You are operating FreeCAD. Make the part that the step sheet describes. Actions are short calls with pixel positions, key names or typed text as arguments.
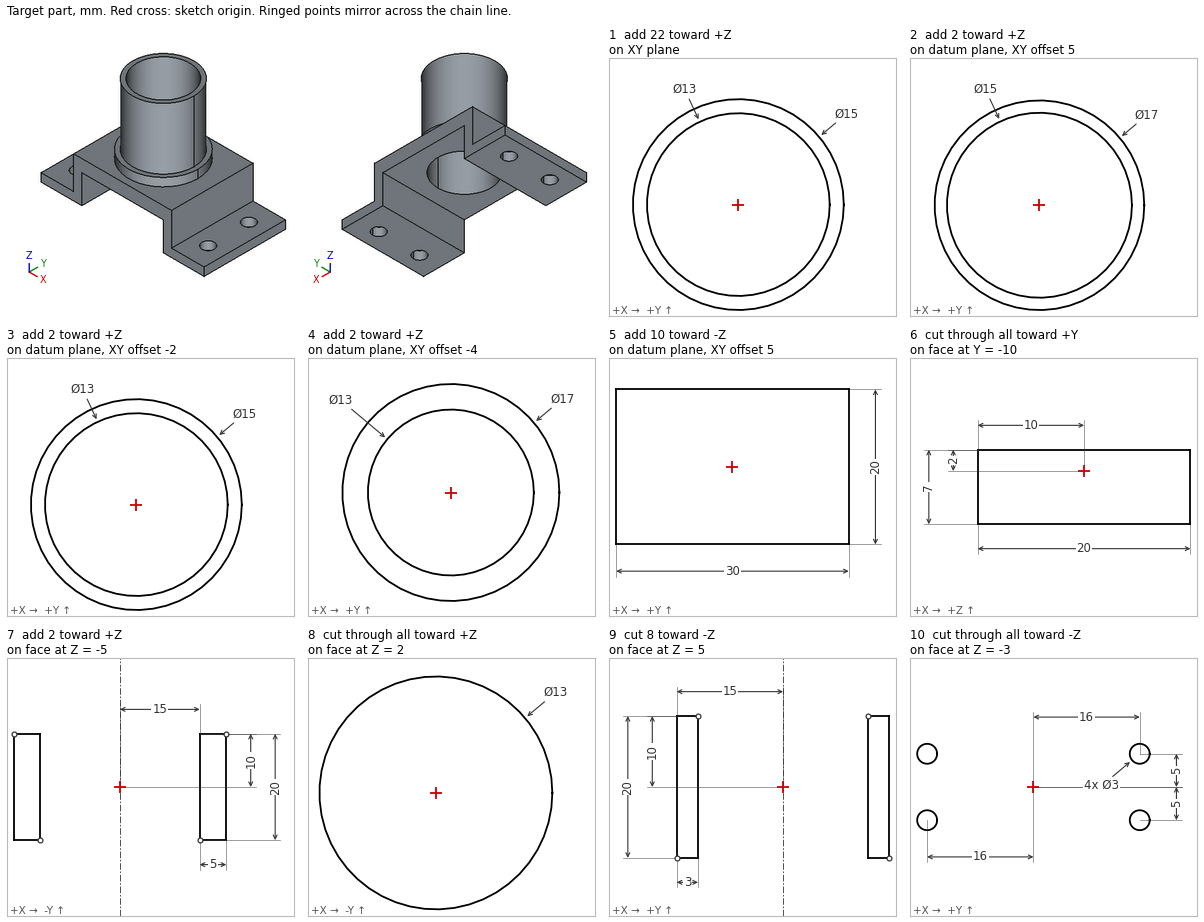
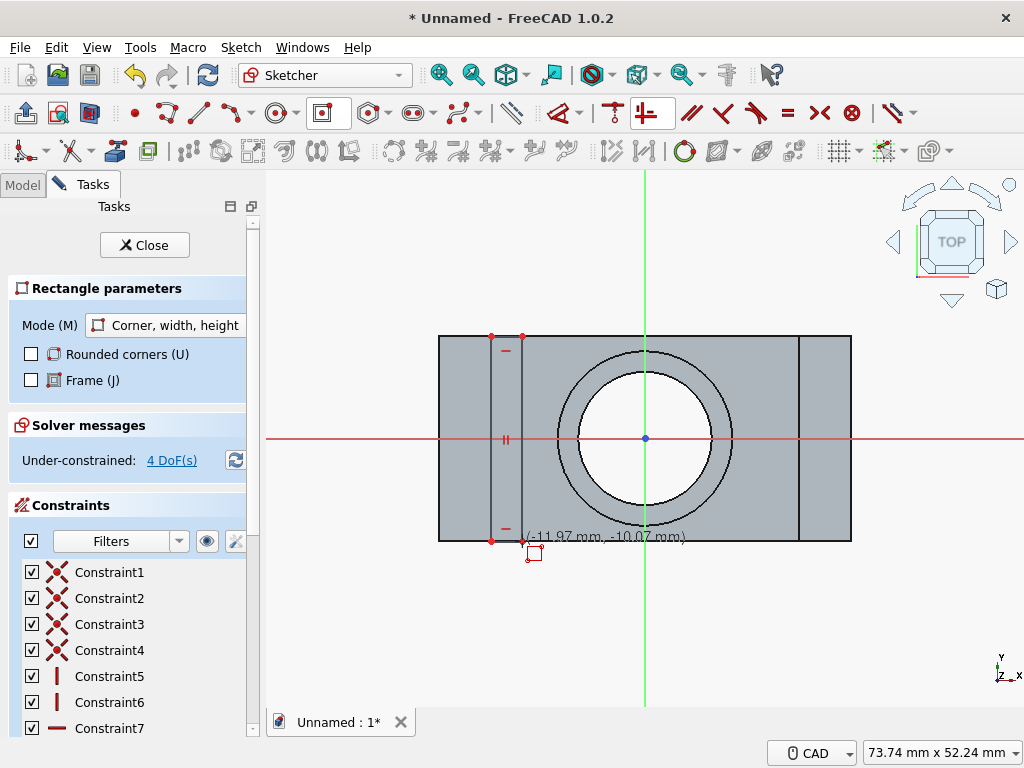
click(768, 336)
click(799, 541)
key(Escape)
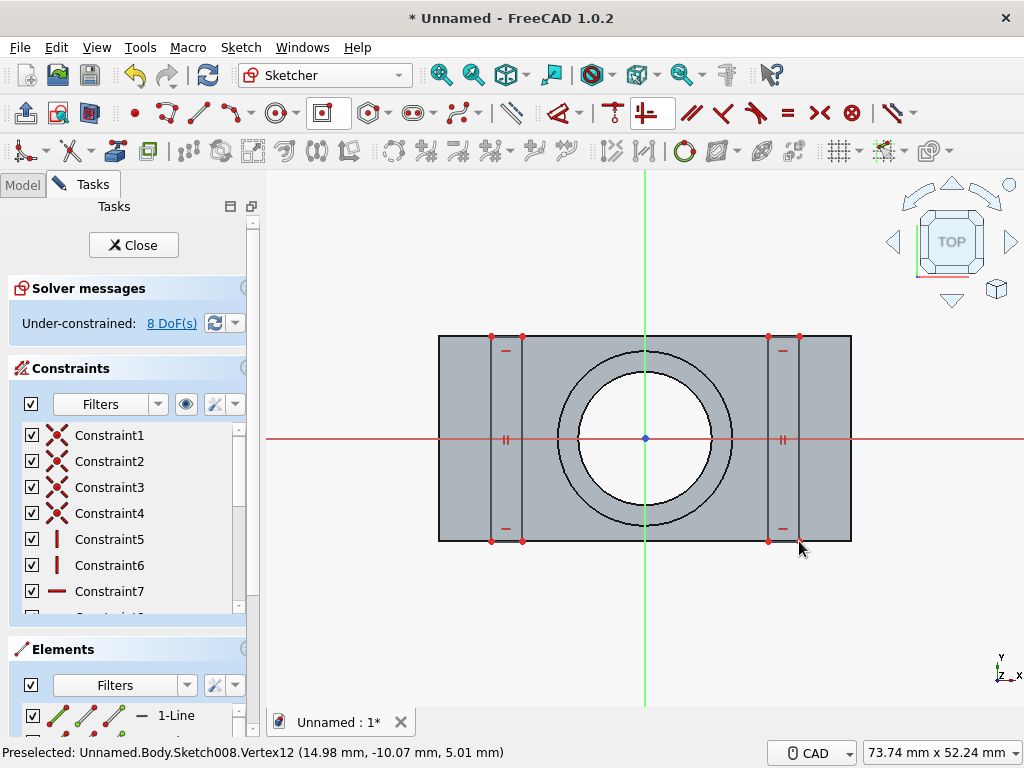
click(522, 337)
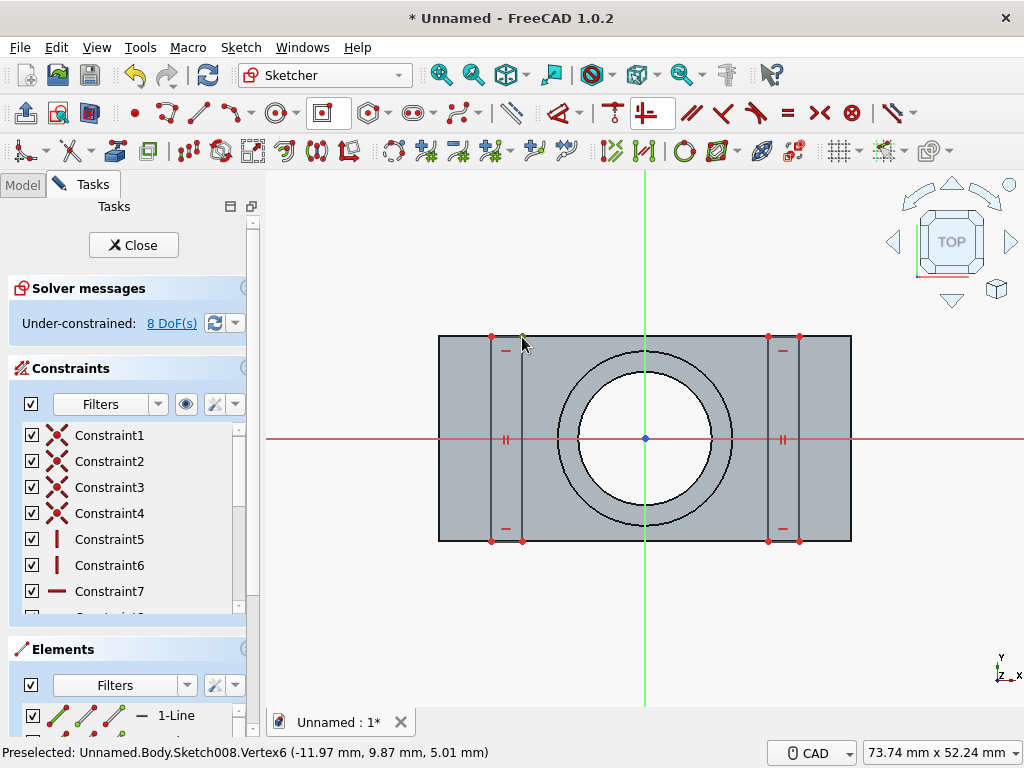
click(768, 337)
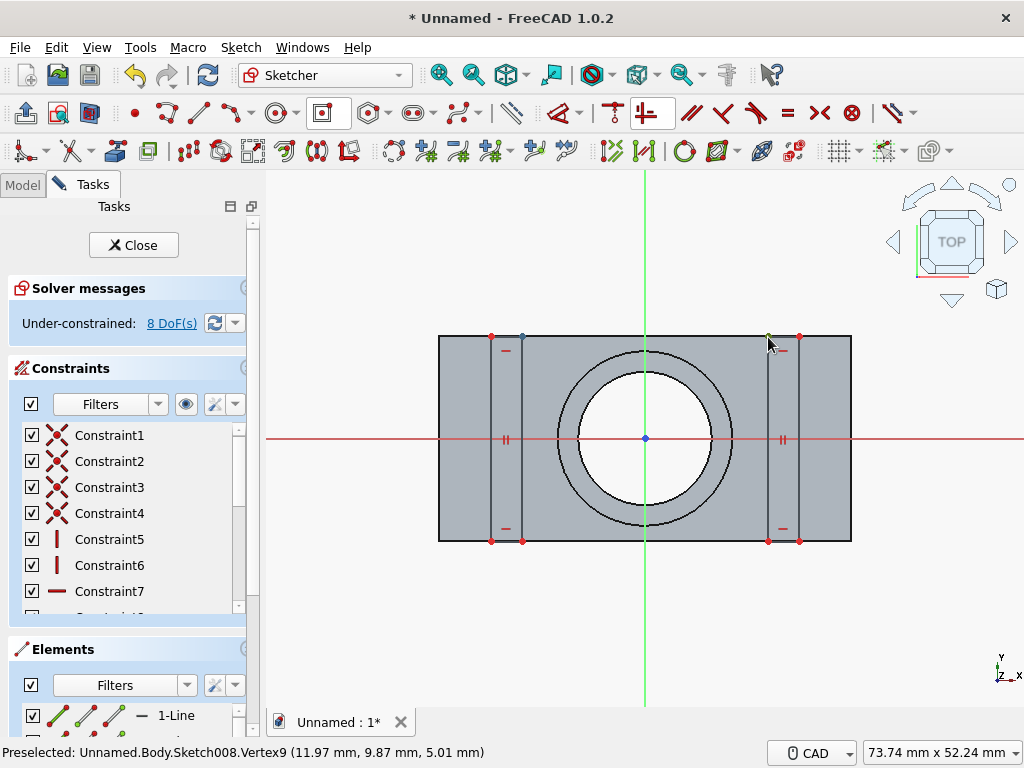
click(645, 645)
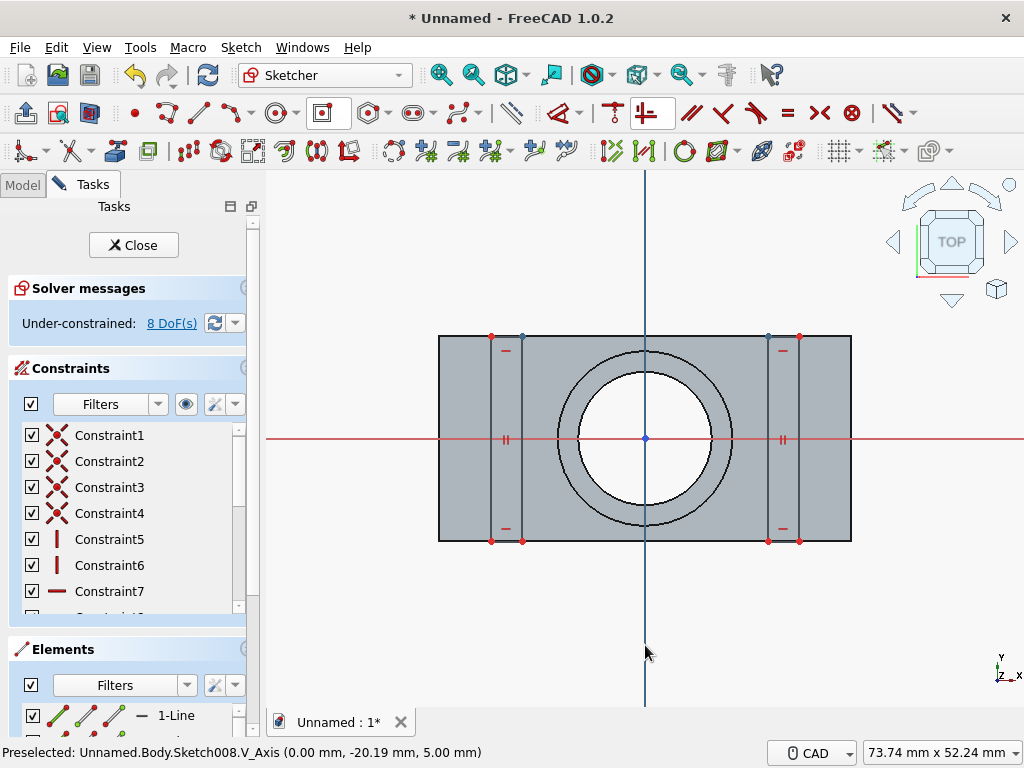
click(820, 114)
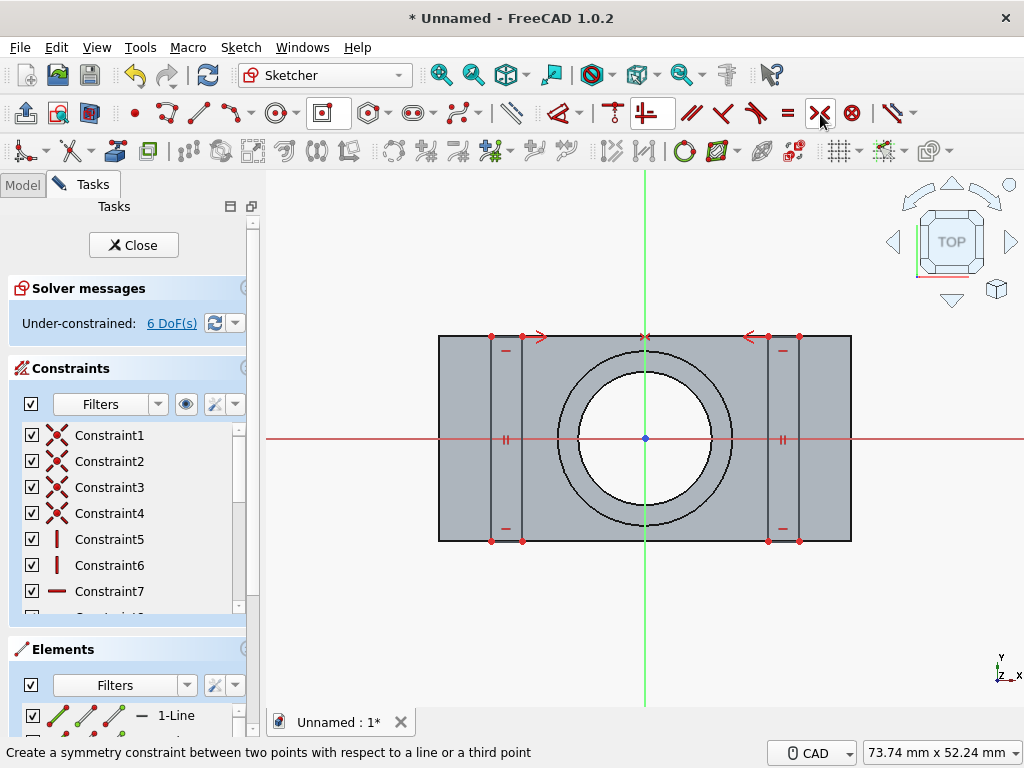
click(491, 542)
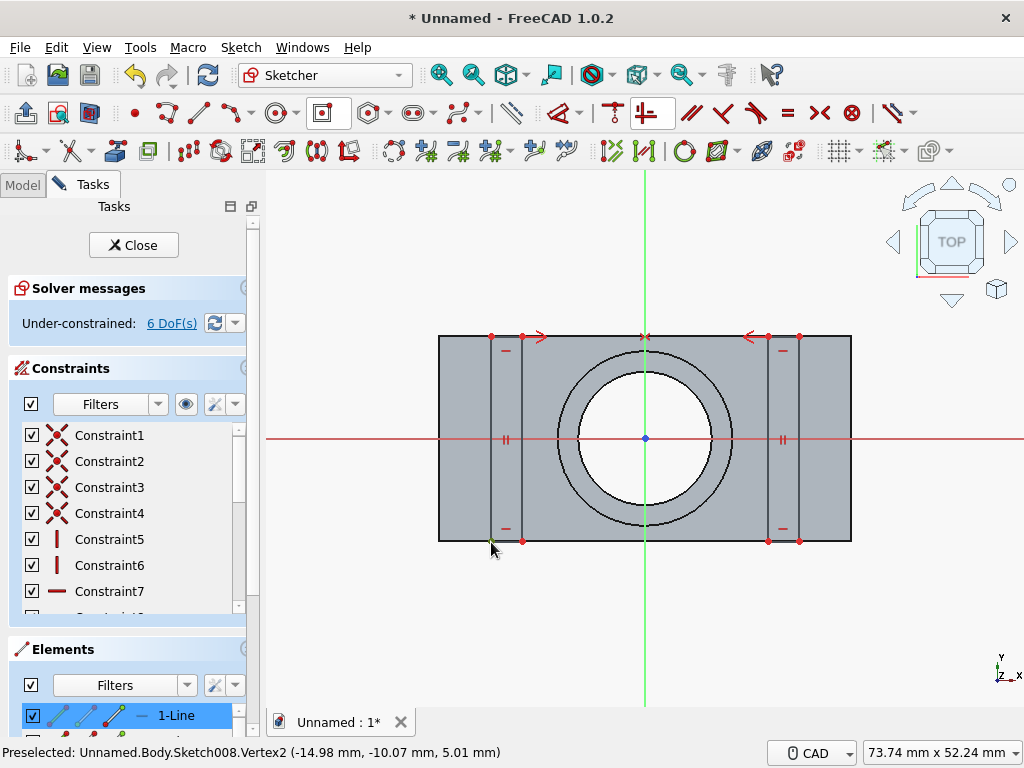
click(799, 542)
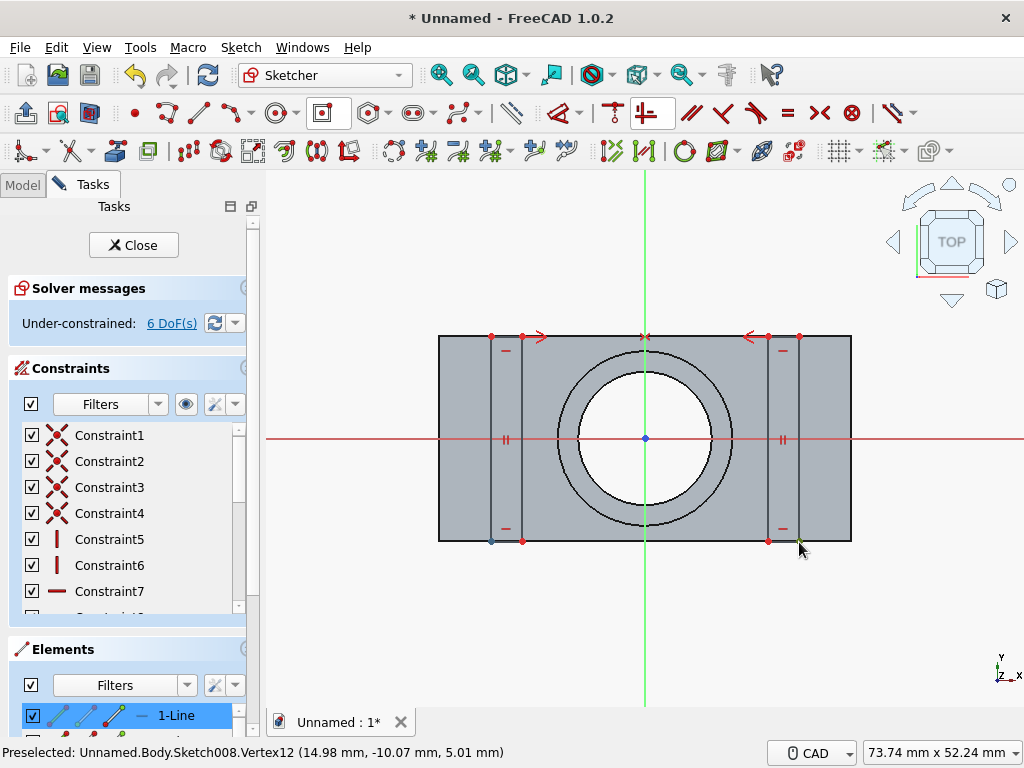
click(645, 645)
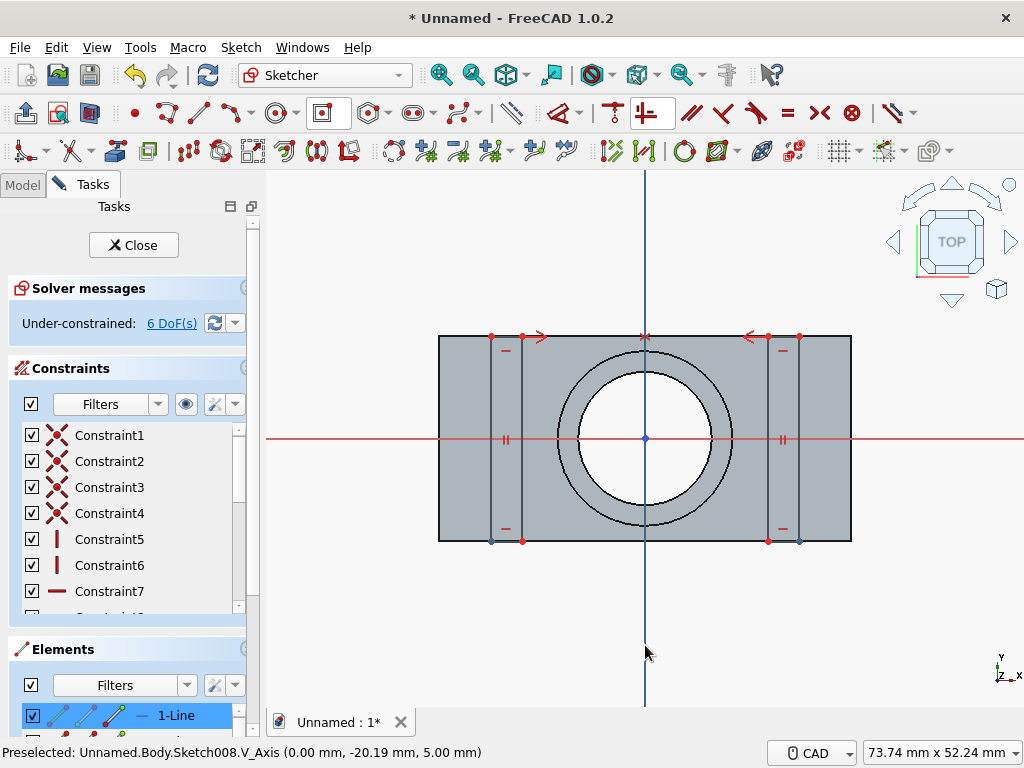
click(820, 114)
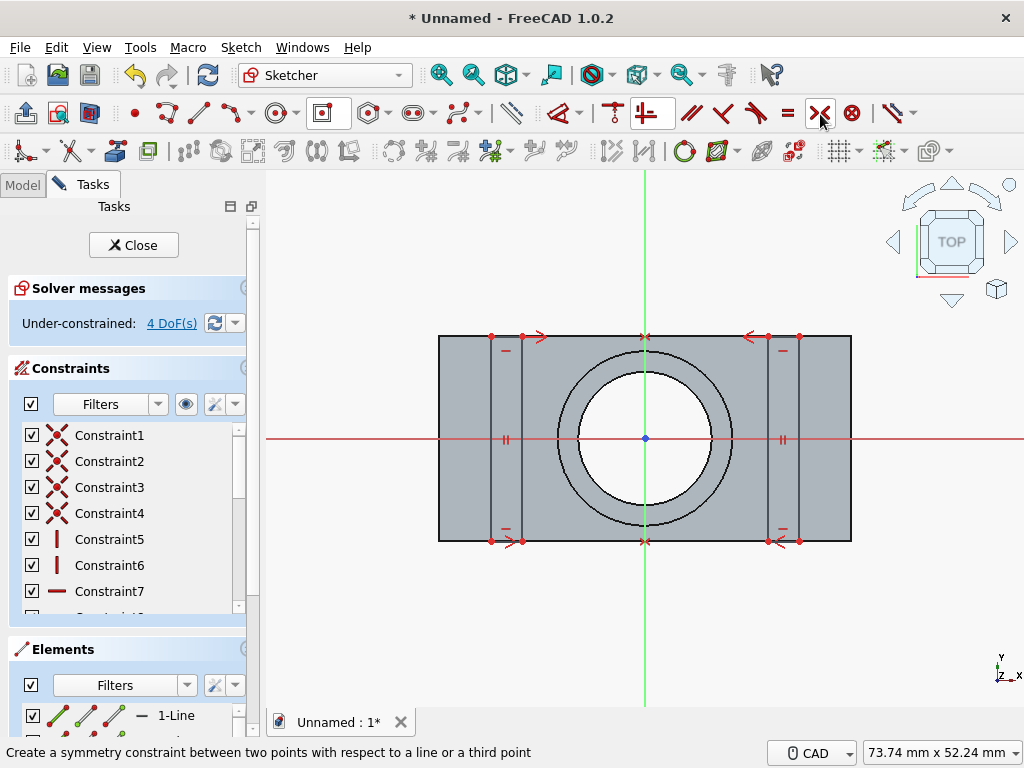
click(558, 114)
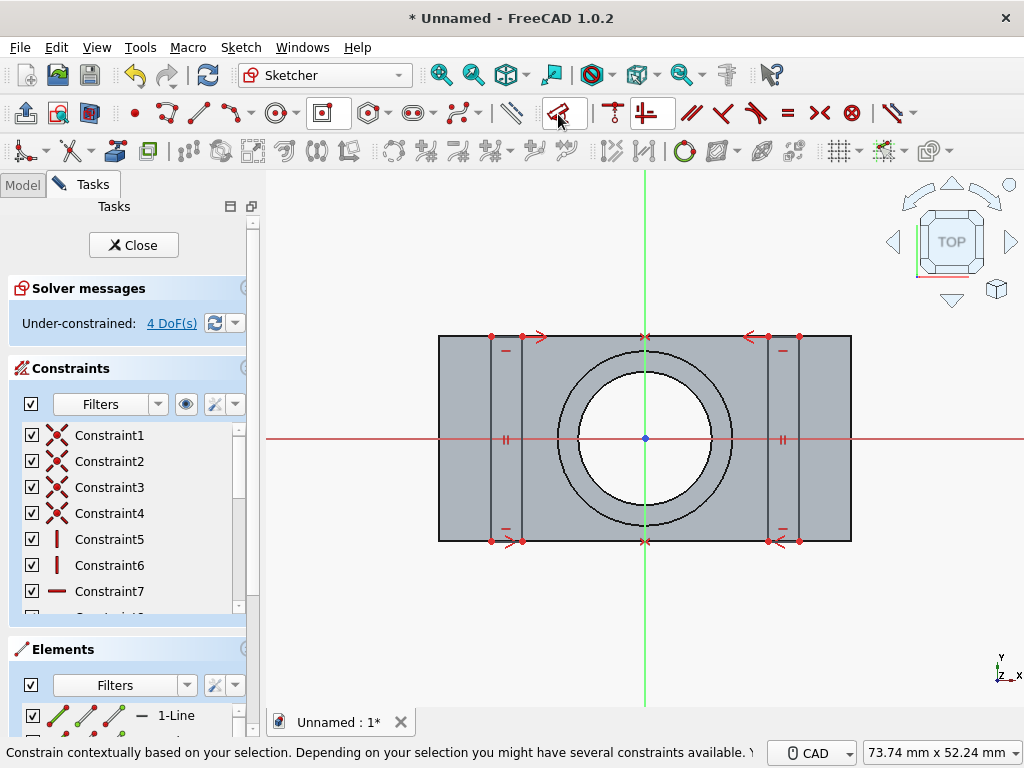
scroll(500, 542, up, 2)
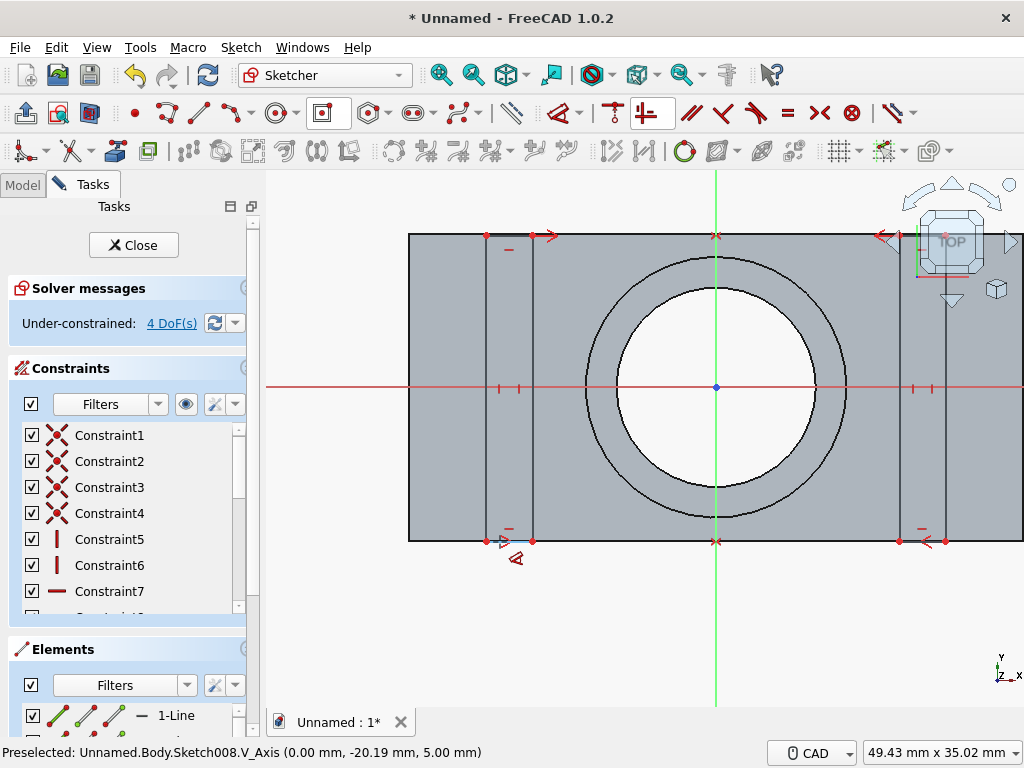
click(500, 542)
click(510, 576)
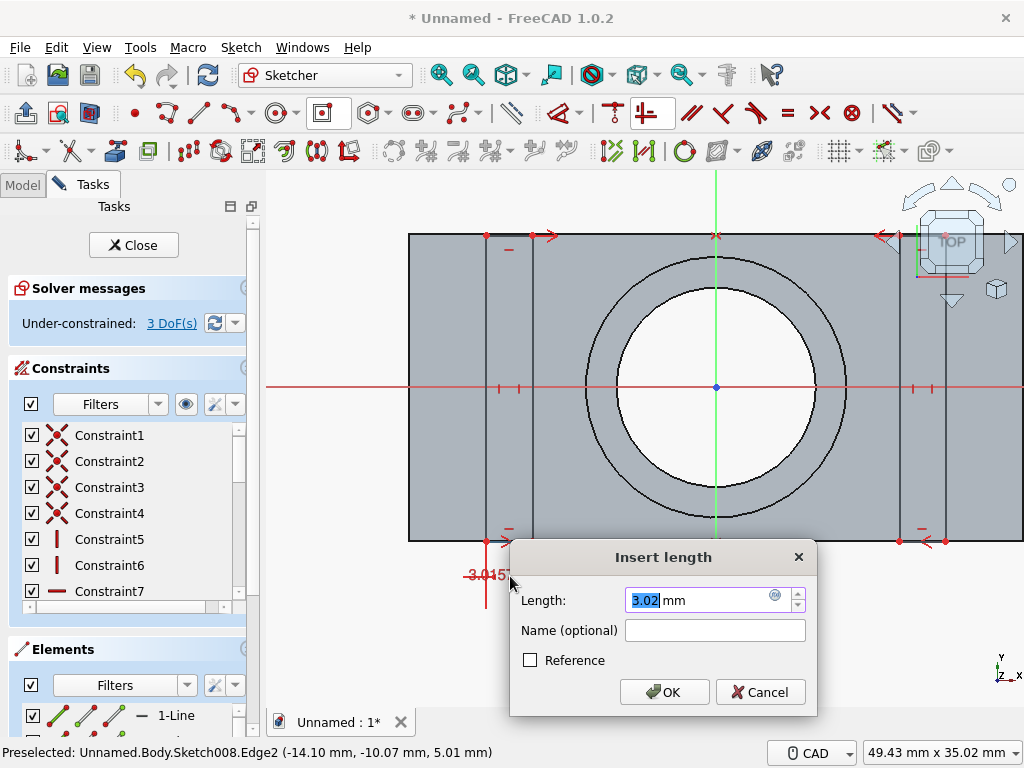
text(3)
key(Return)